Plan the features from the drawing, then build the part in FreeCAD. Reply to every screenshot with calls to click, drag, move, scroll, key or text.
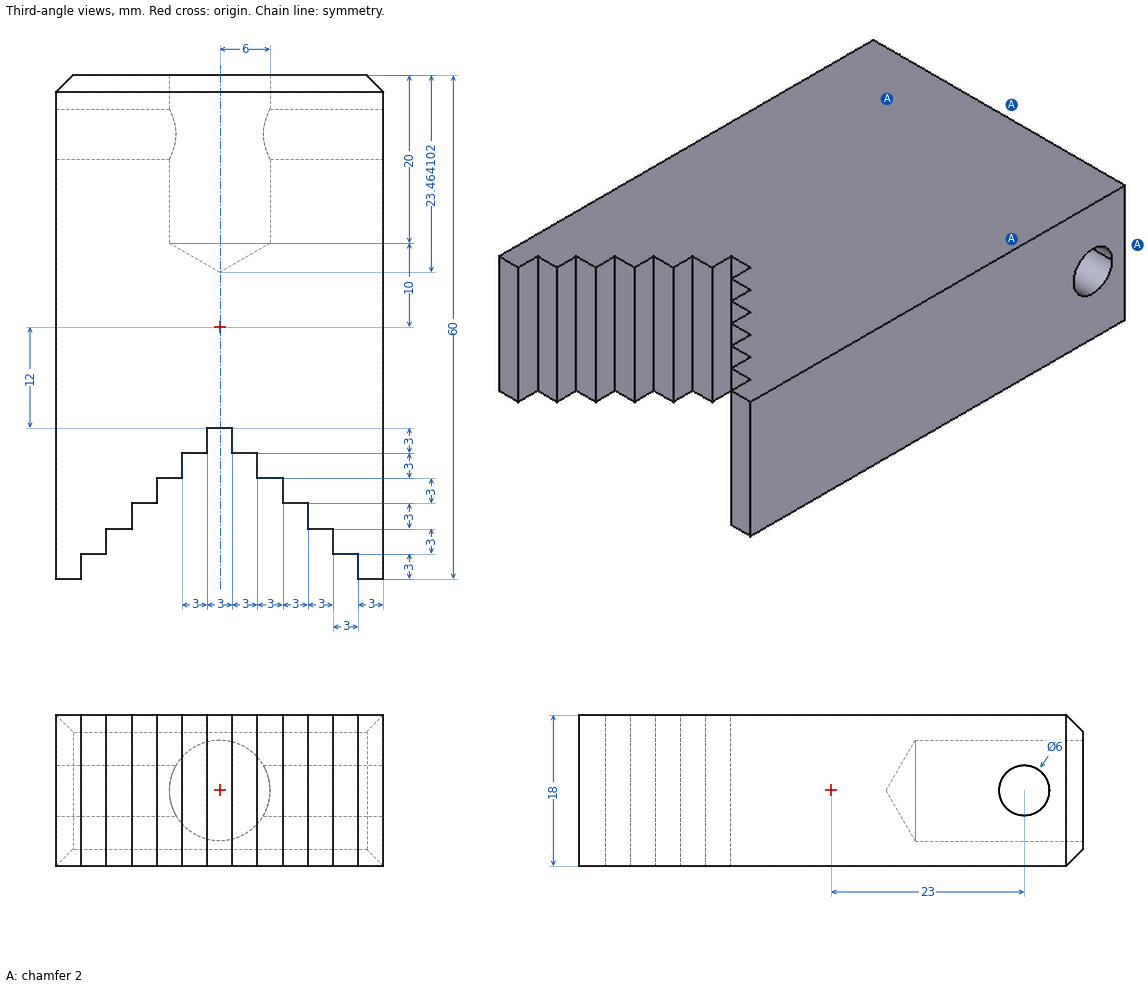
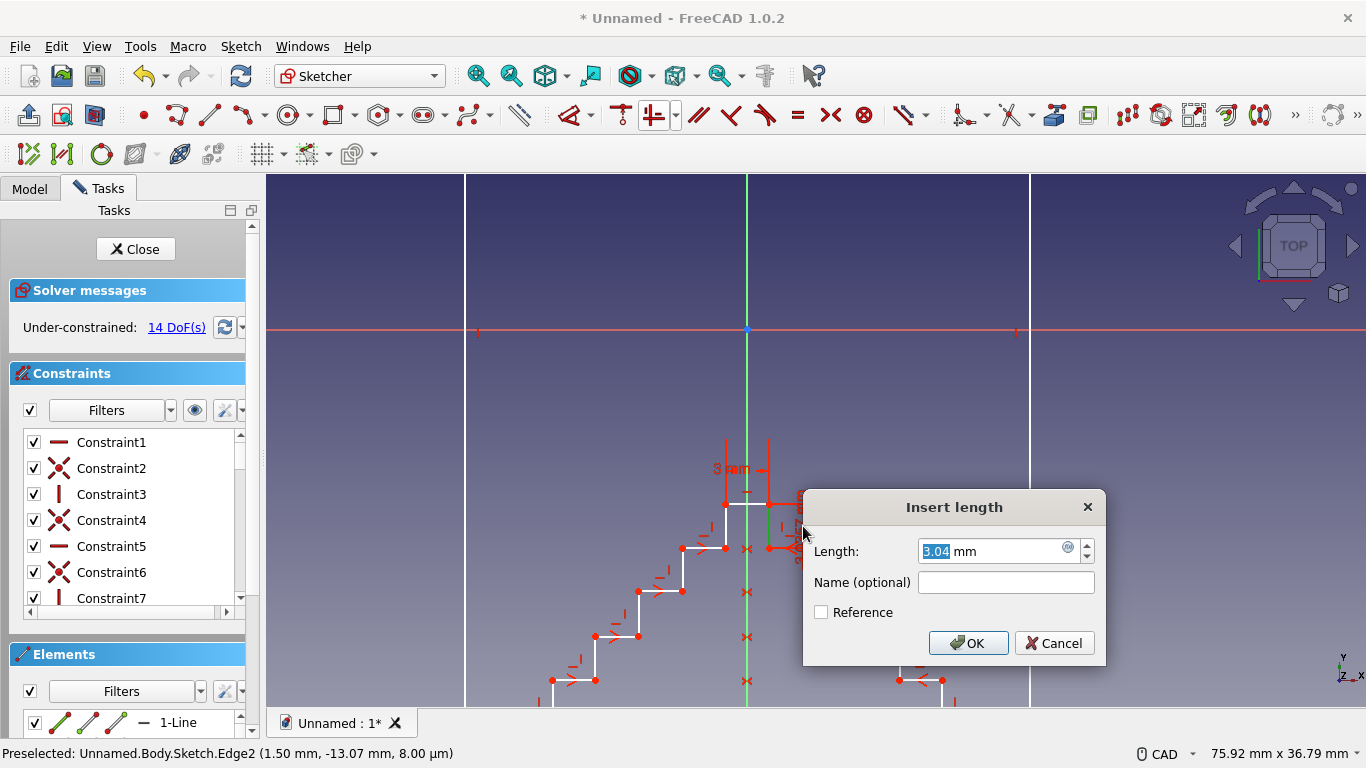
text(3)
key(Return)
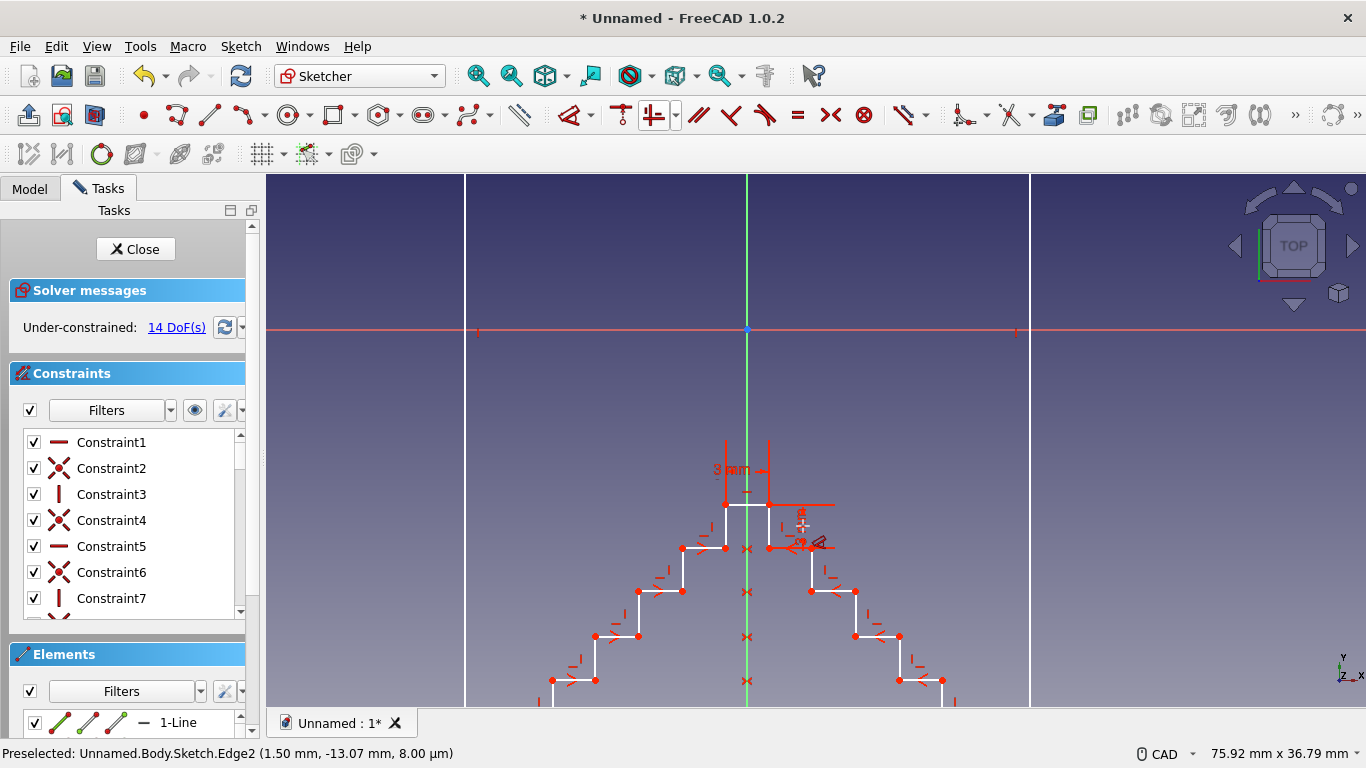
click(782, 548)
click(790, 582)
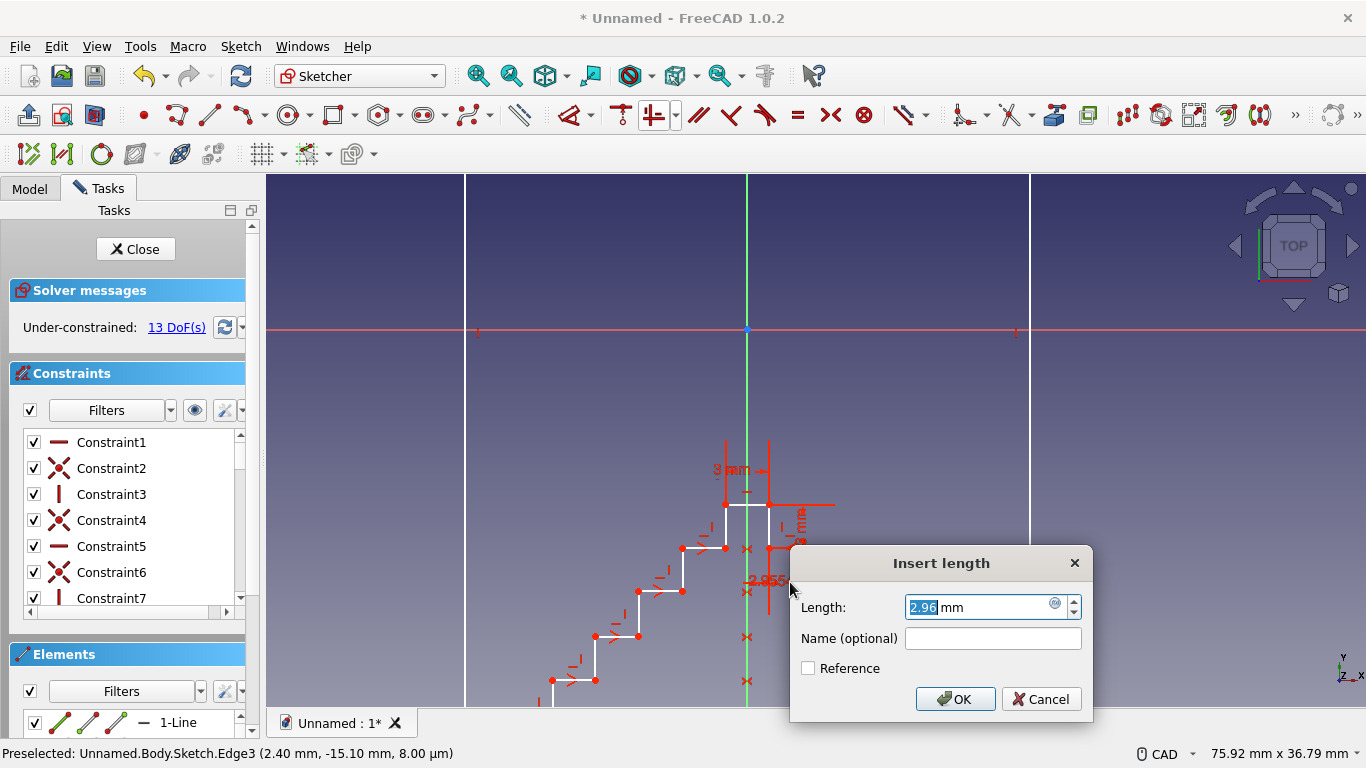
text(3)
key(Return)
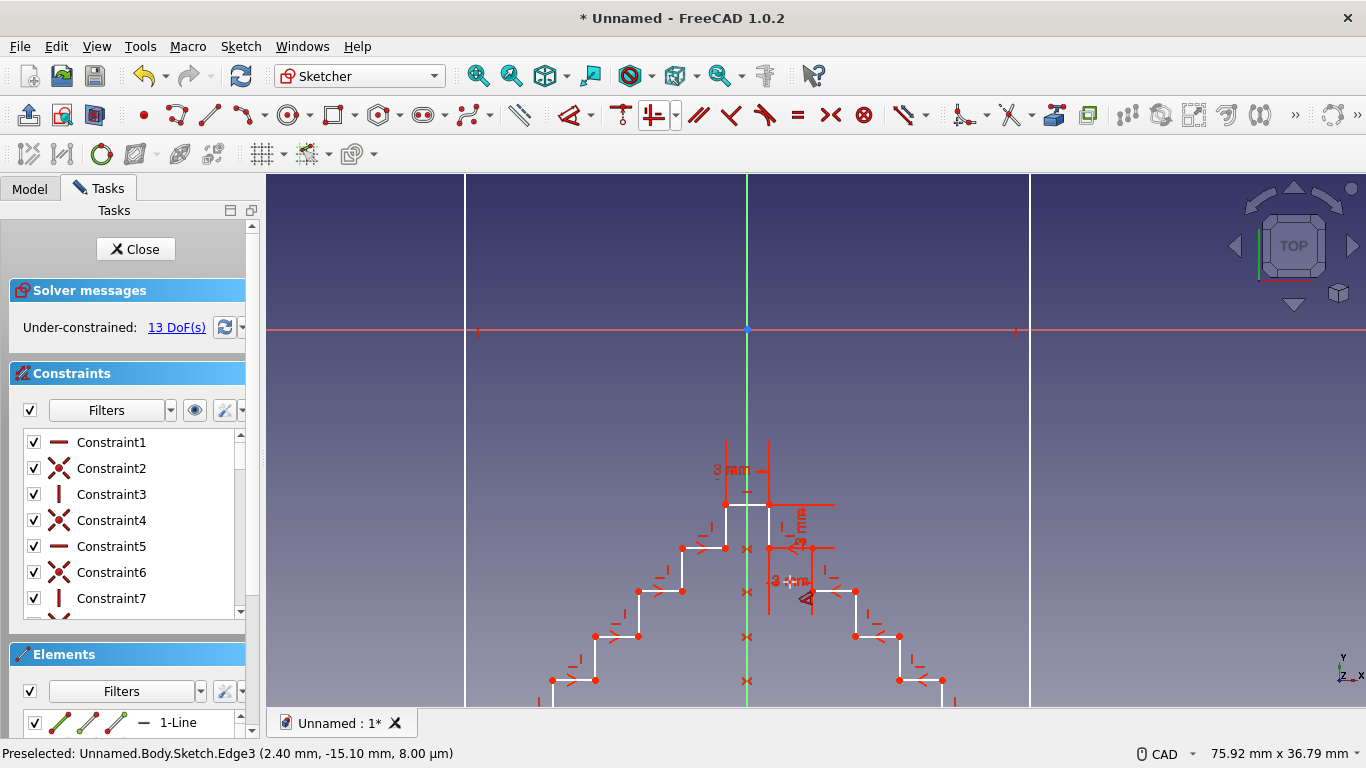
click(812, 561)
click(846, 560)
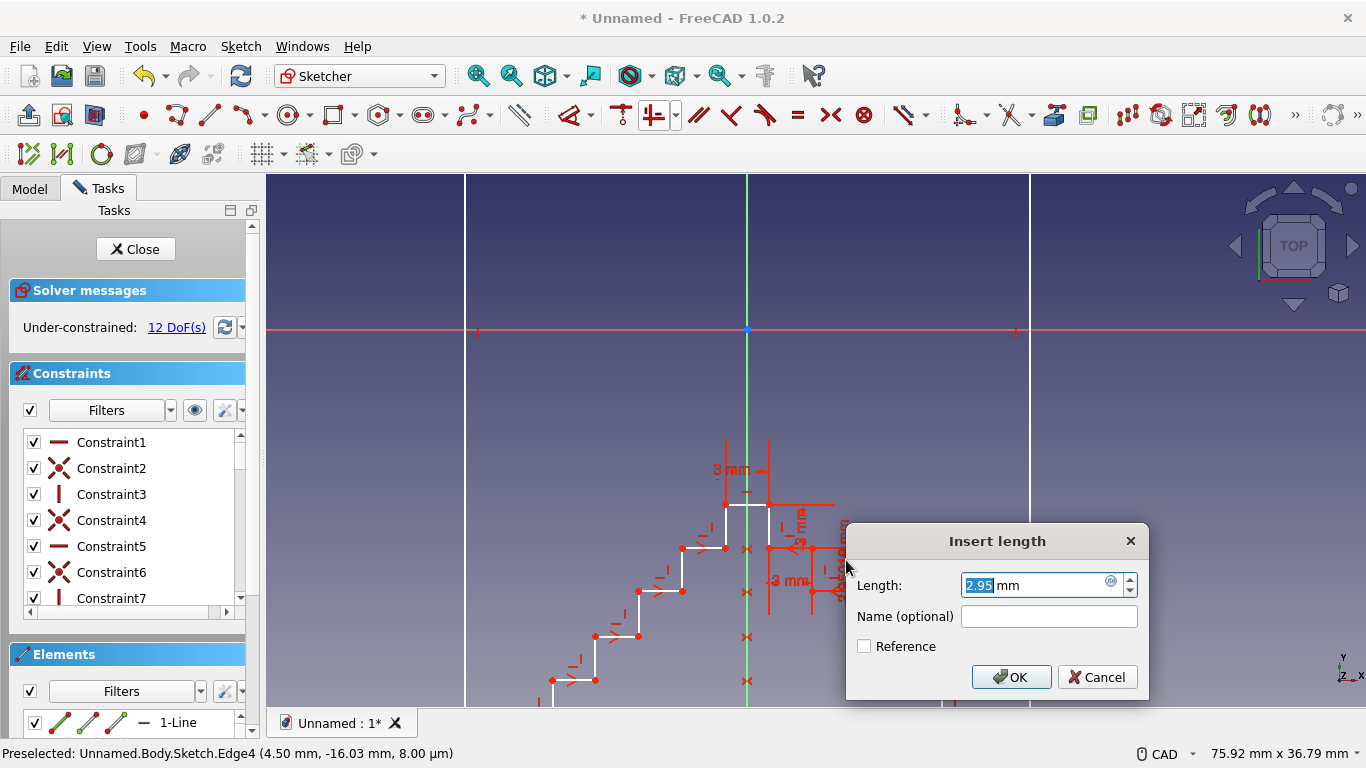
text(3)
key(Return)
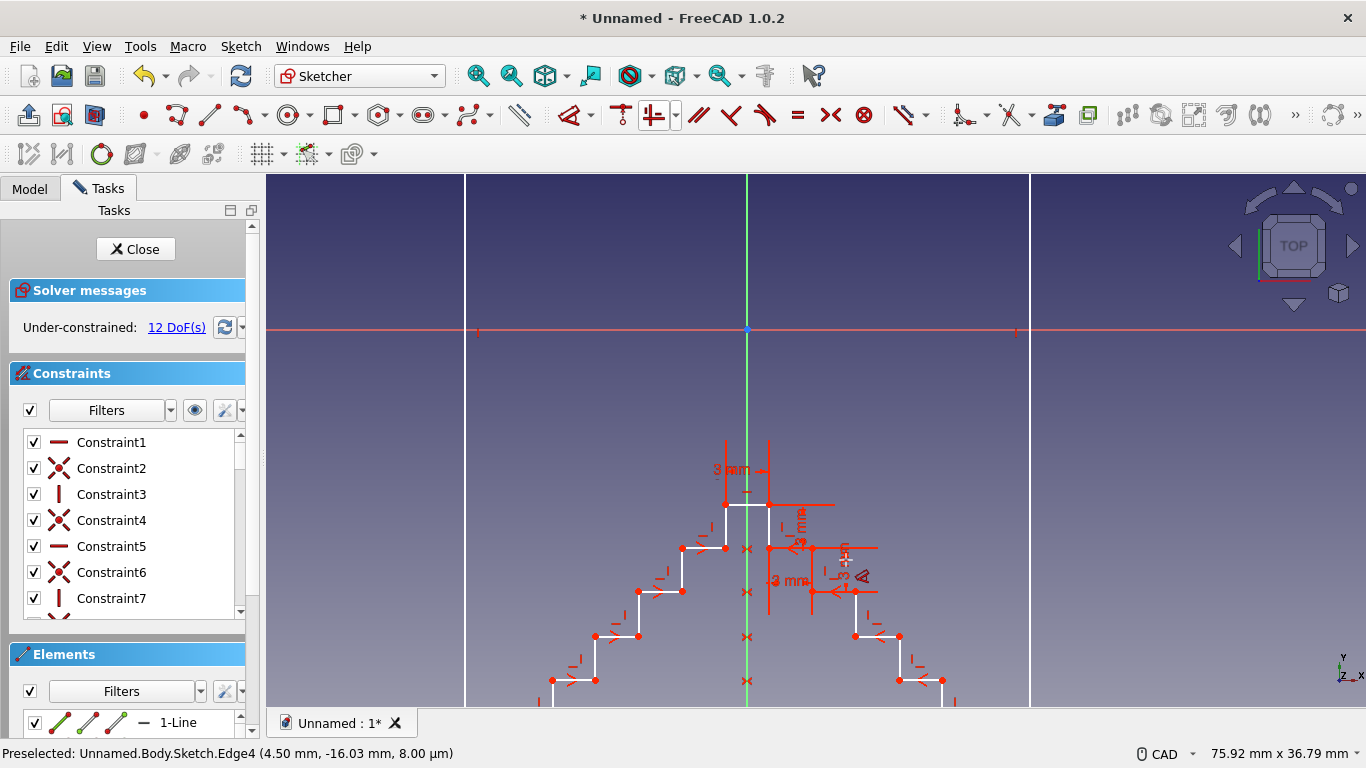
click(825, 592)
click(834, 626)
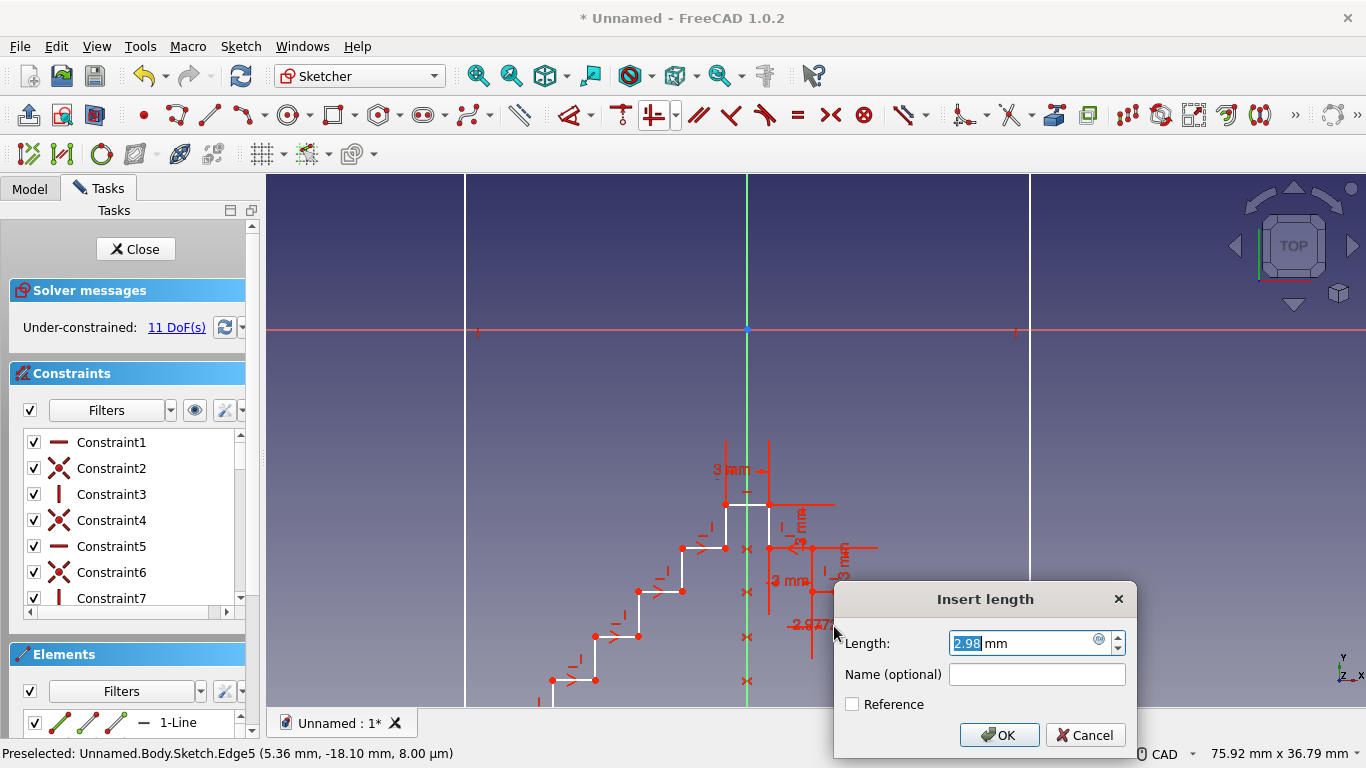
text(3)
key(Return)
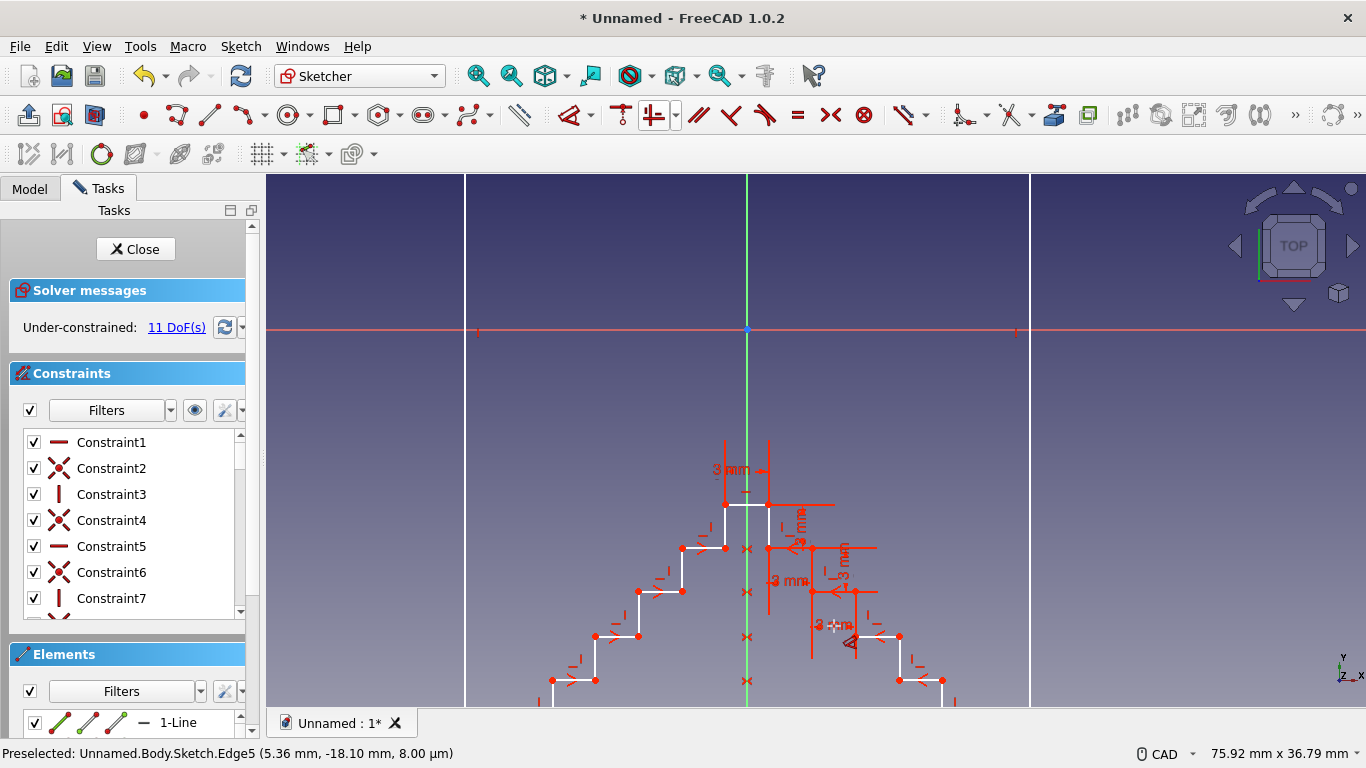
click(856, 605)
click(890, 604)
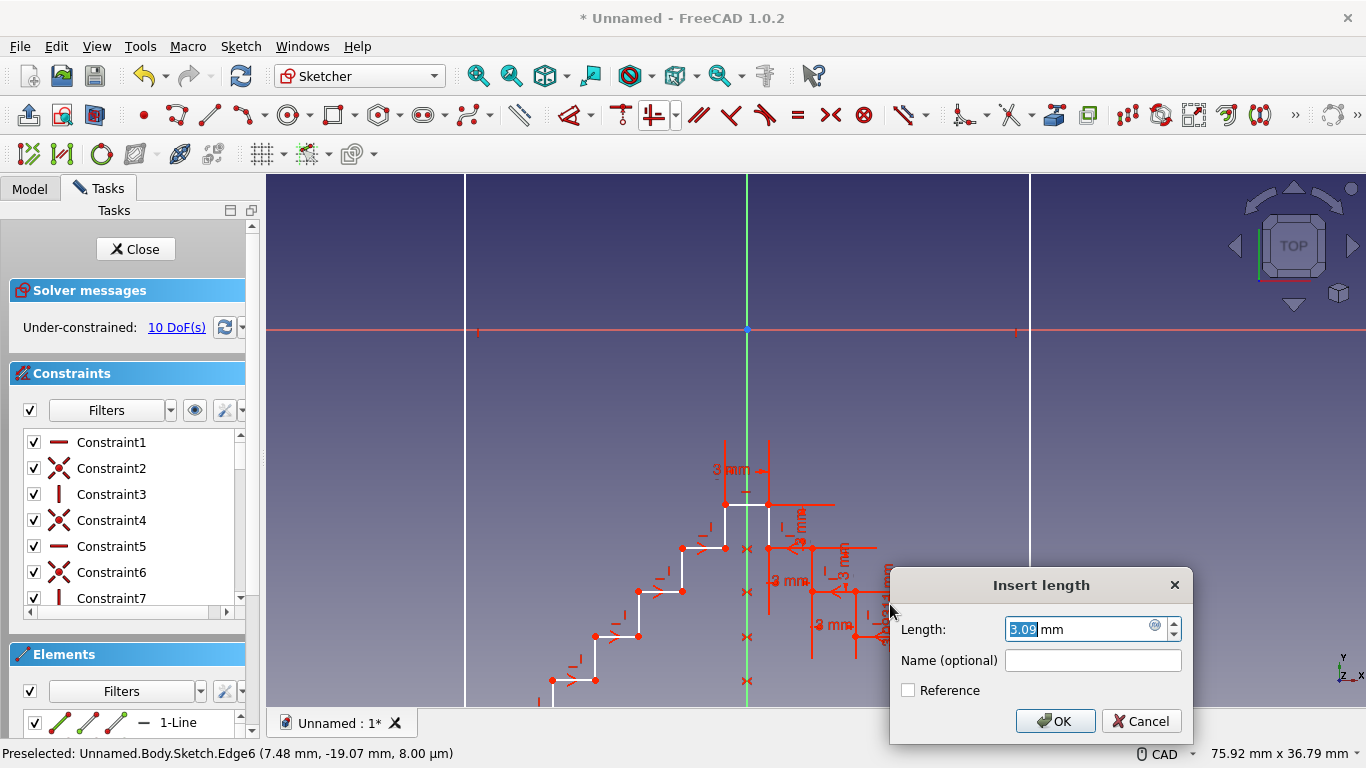
text(3)
key(Return)